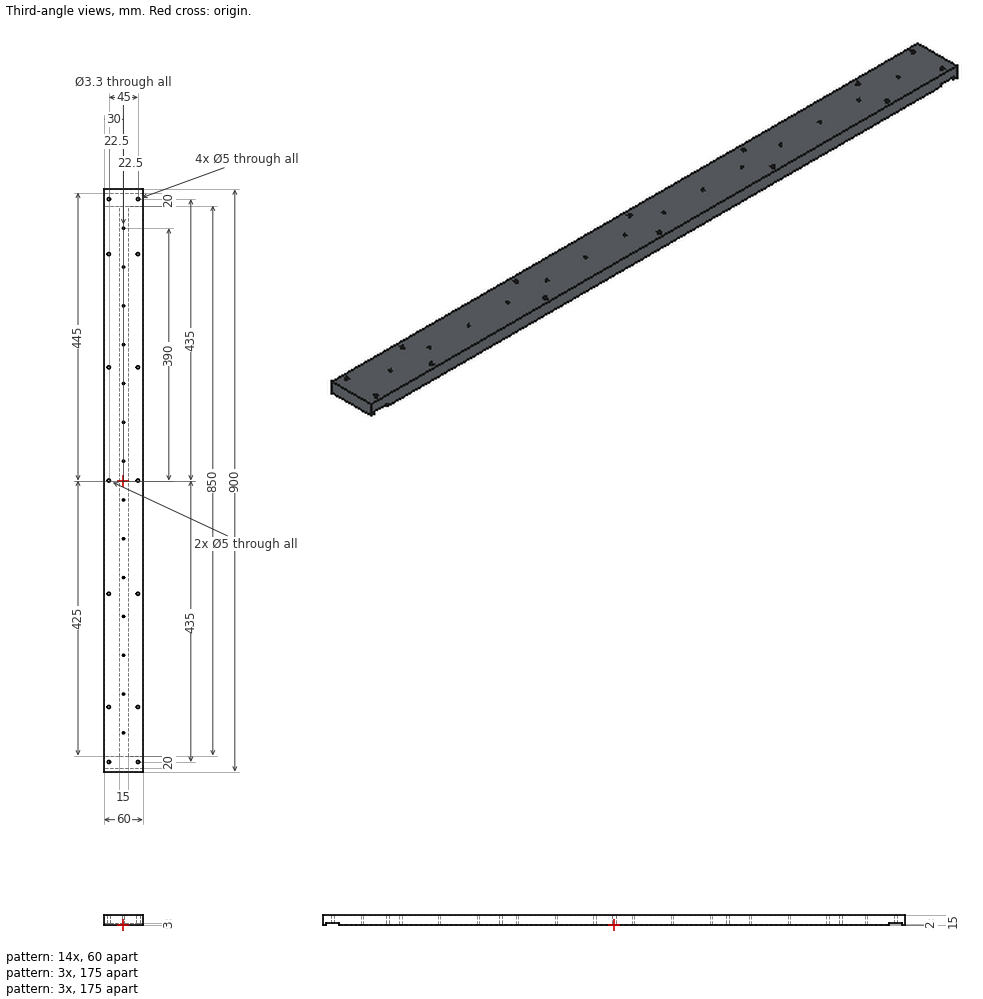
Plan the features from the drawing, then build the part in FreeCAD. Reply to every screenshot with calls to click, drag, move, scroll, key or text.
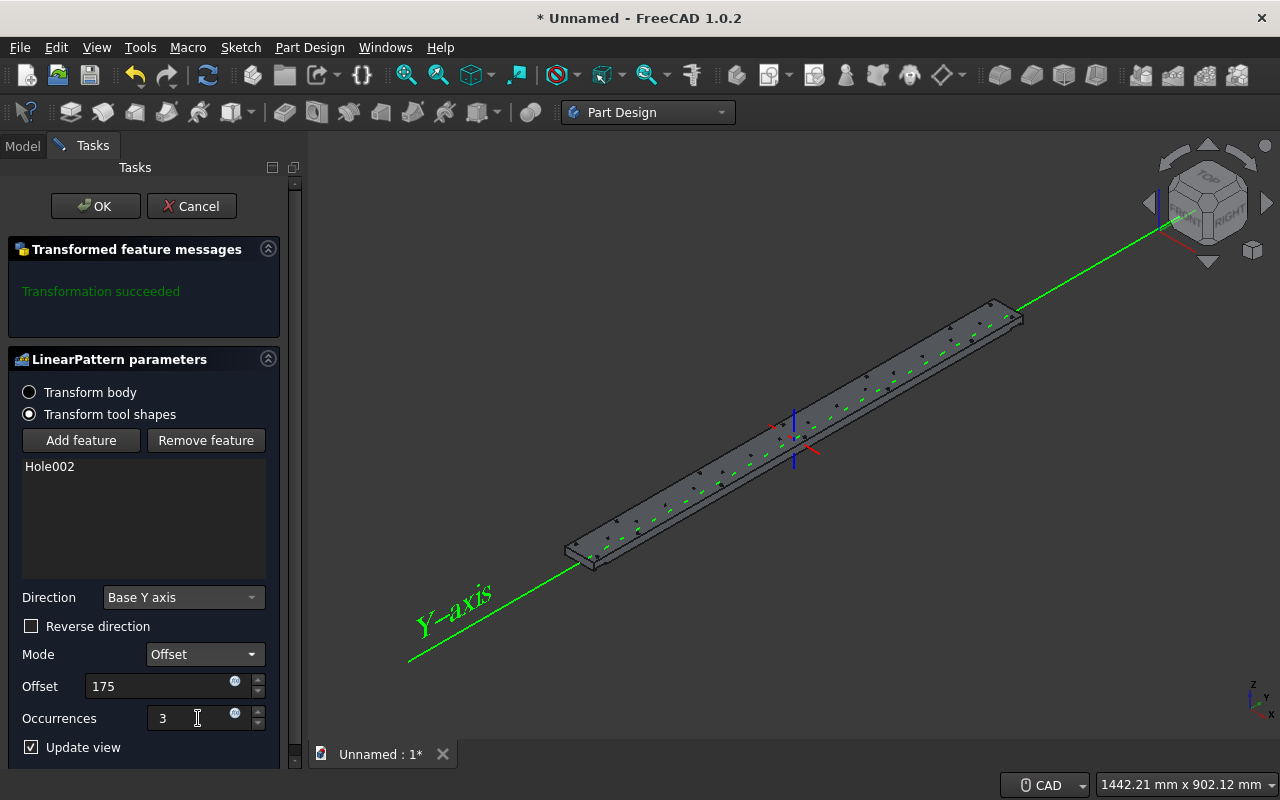
click(96, 206)